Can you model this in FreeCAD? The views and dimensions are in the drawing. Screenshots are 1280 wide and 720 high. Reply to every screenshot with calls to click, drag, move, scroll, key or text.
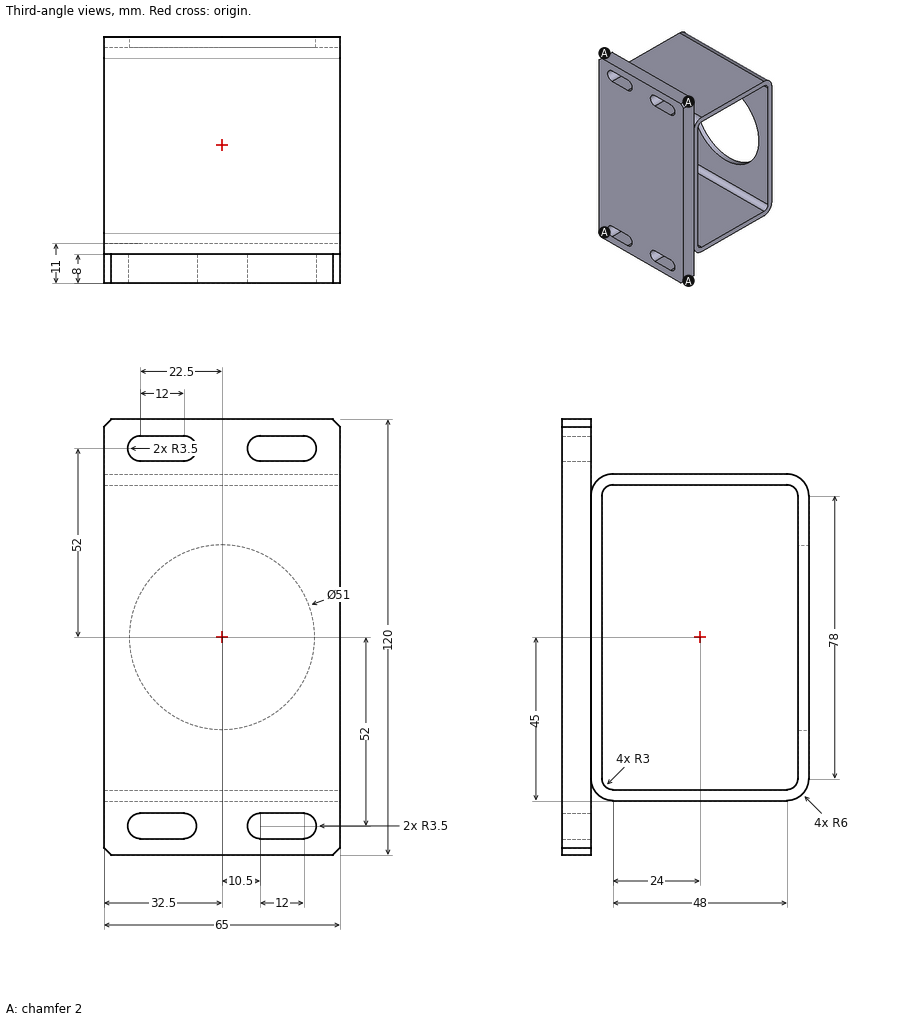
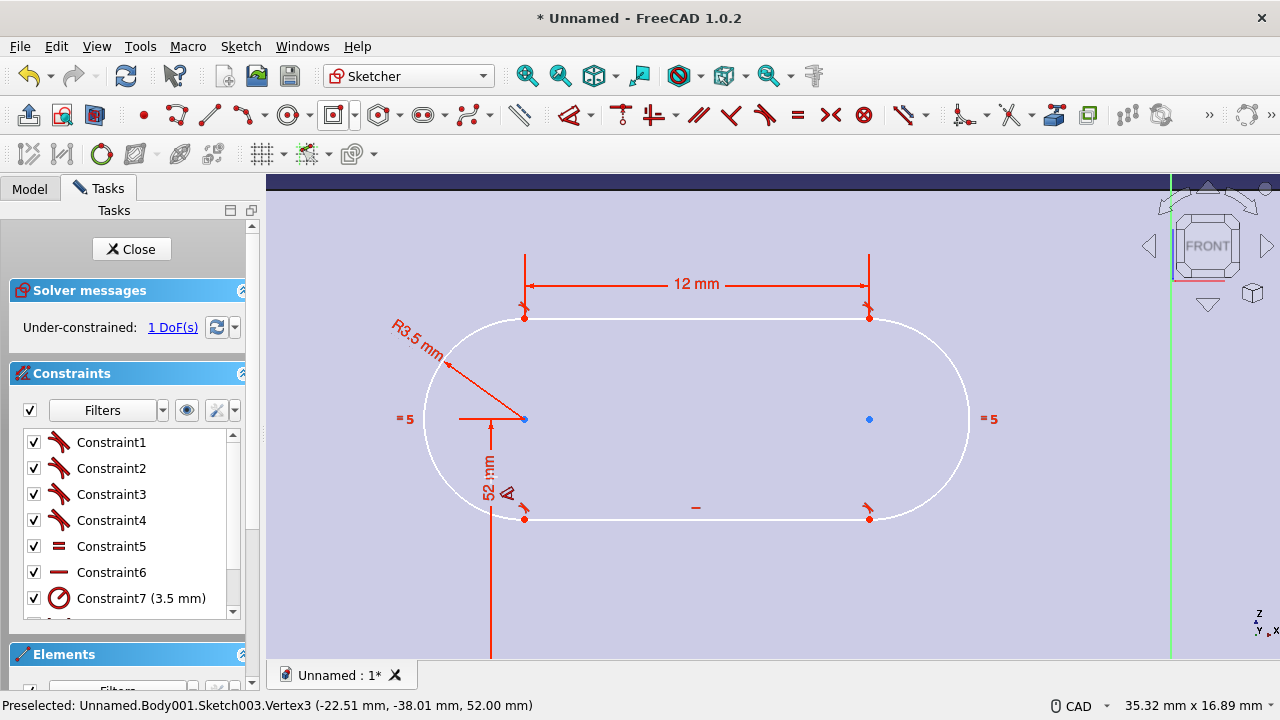
click(525, 319)
click(820, 285)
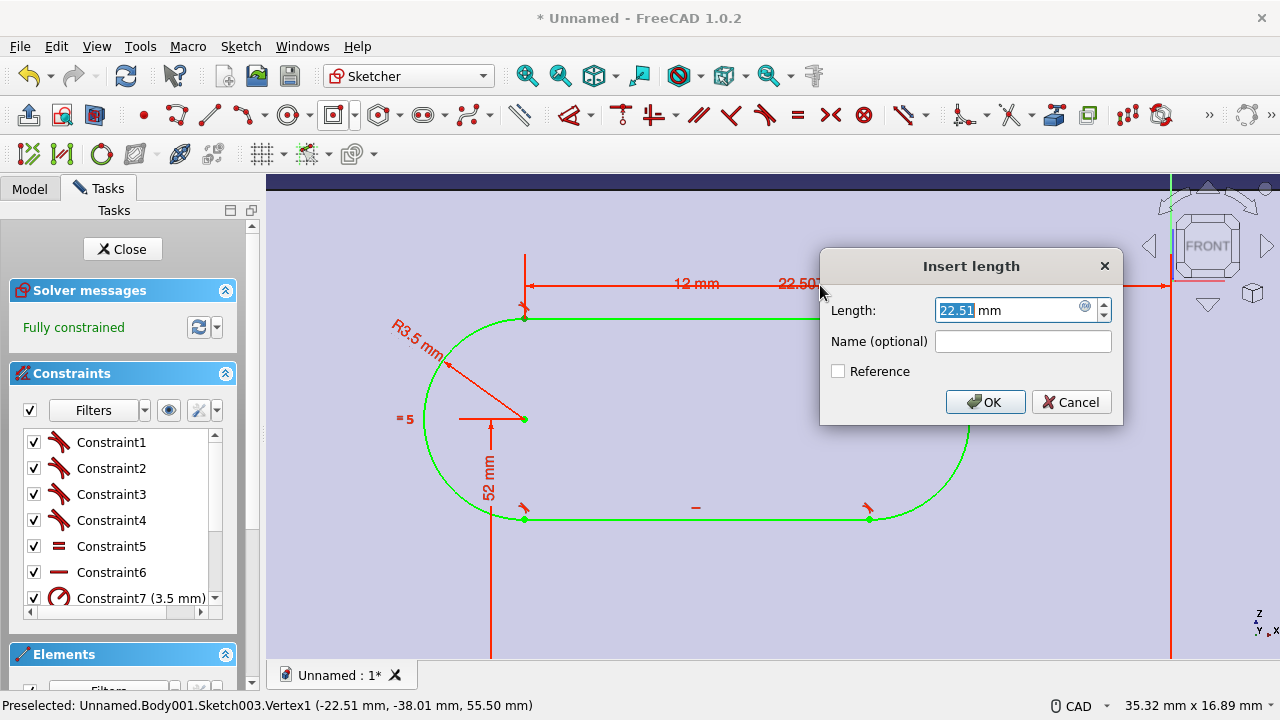
text(22.5)
key(Return)
key(Escape)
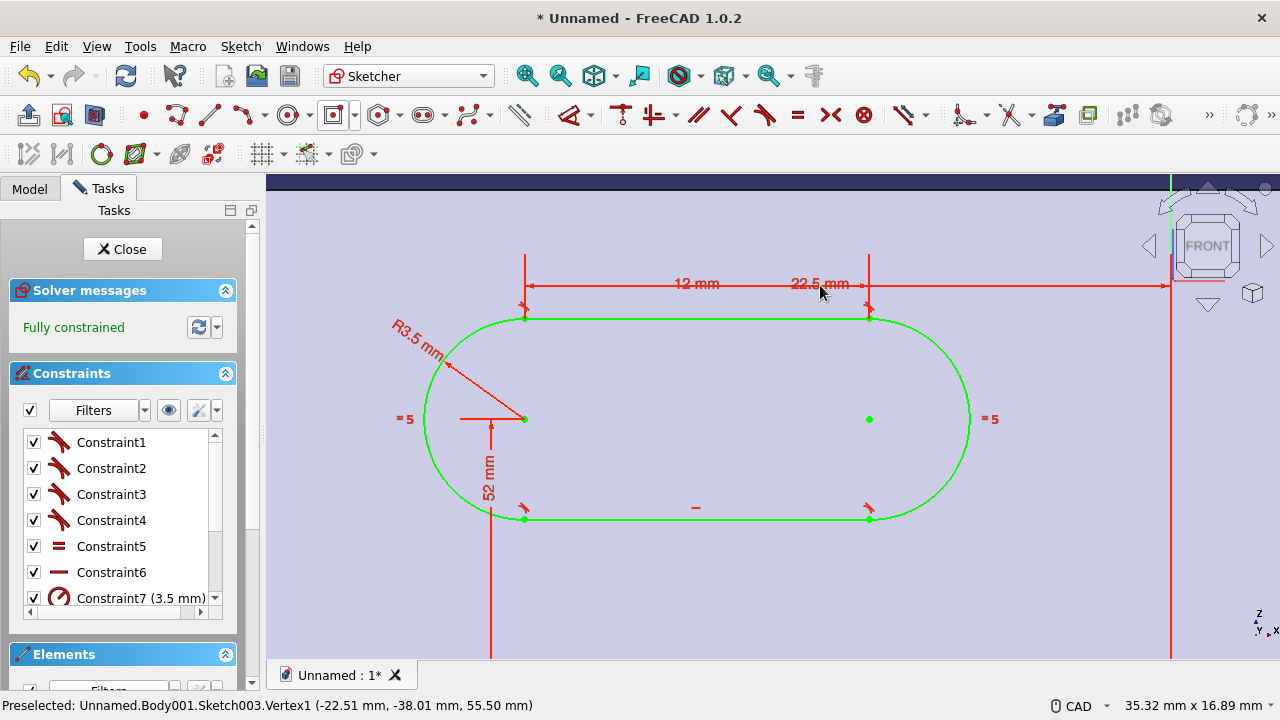
click(123, 249)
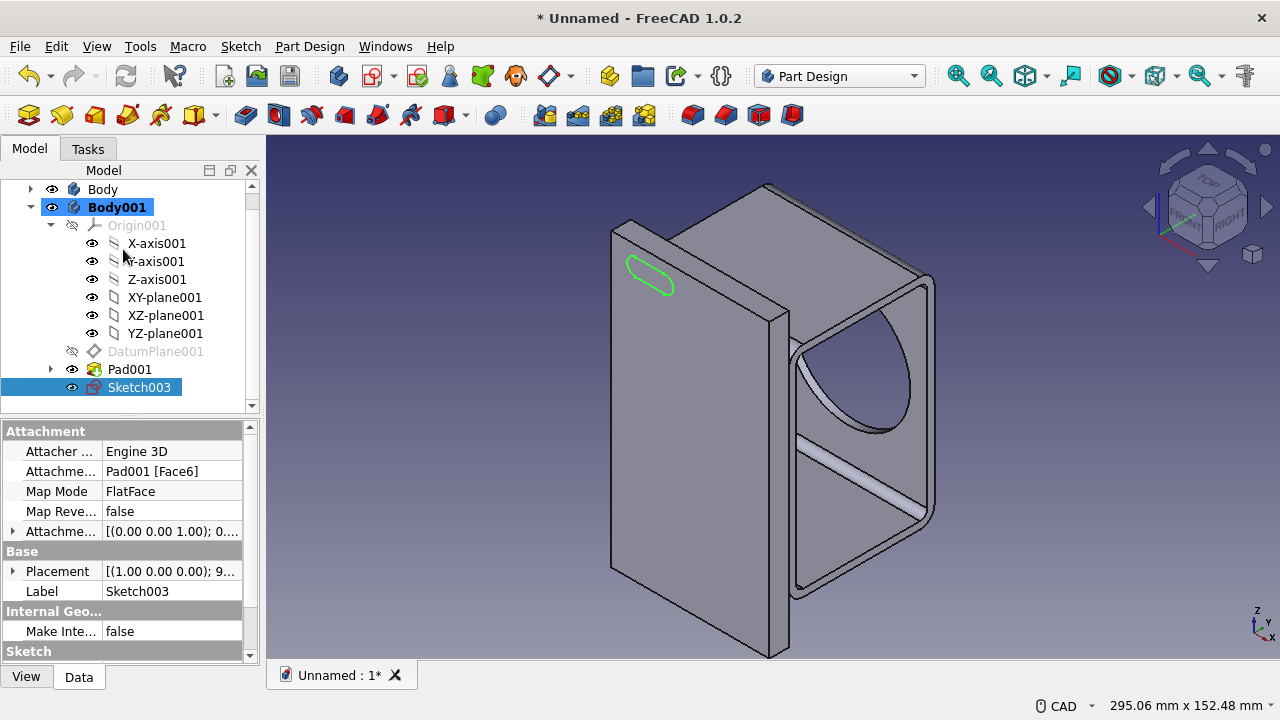
click(246, 116)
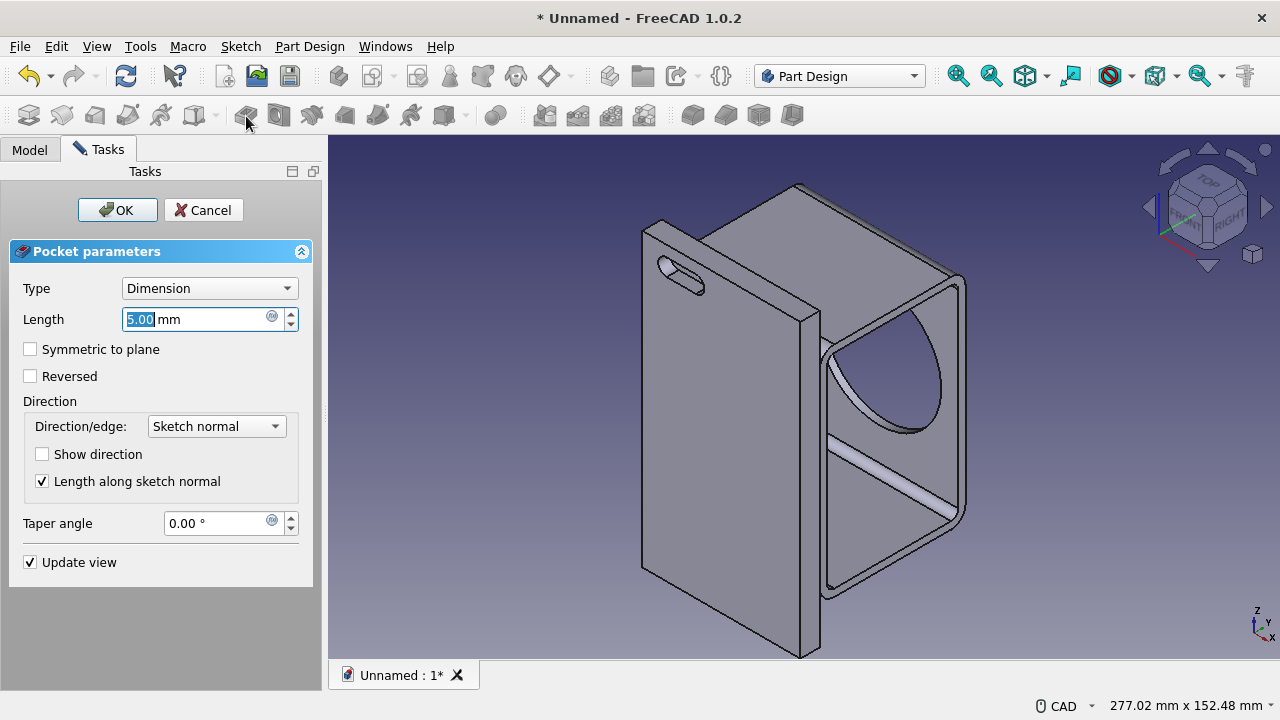
text(11)
key(Tab)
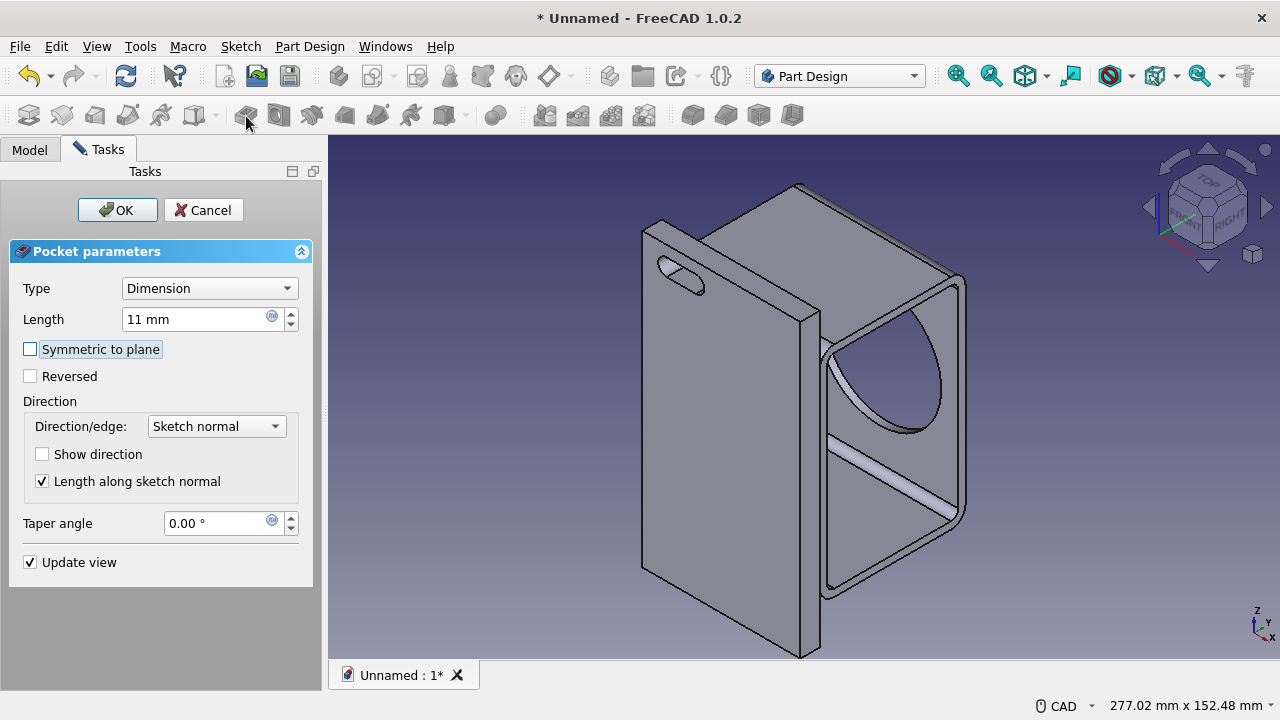
click(118, 210)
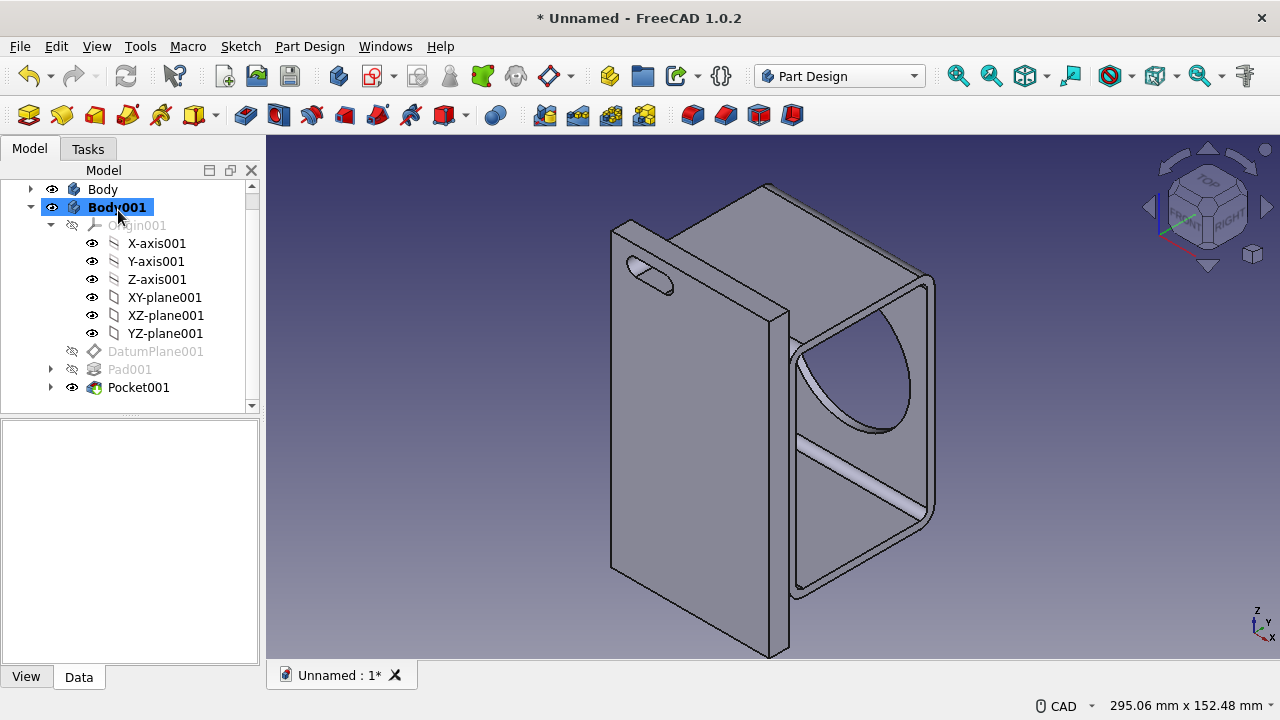
click(117, 387)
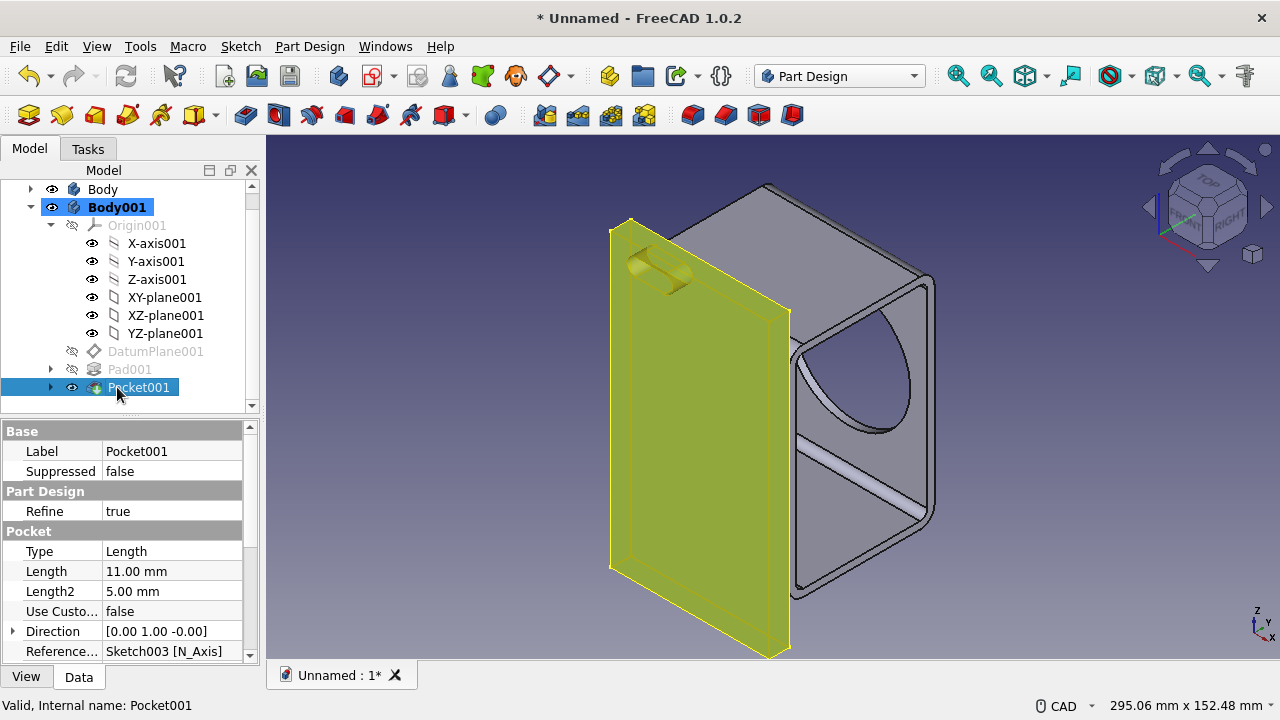
click(545, 116)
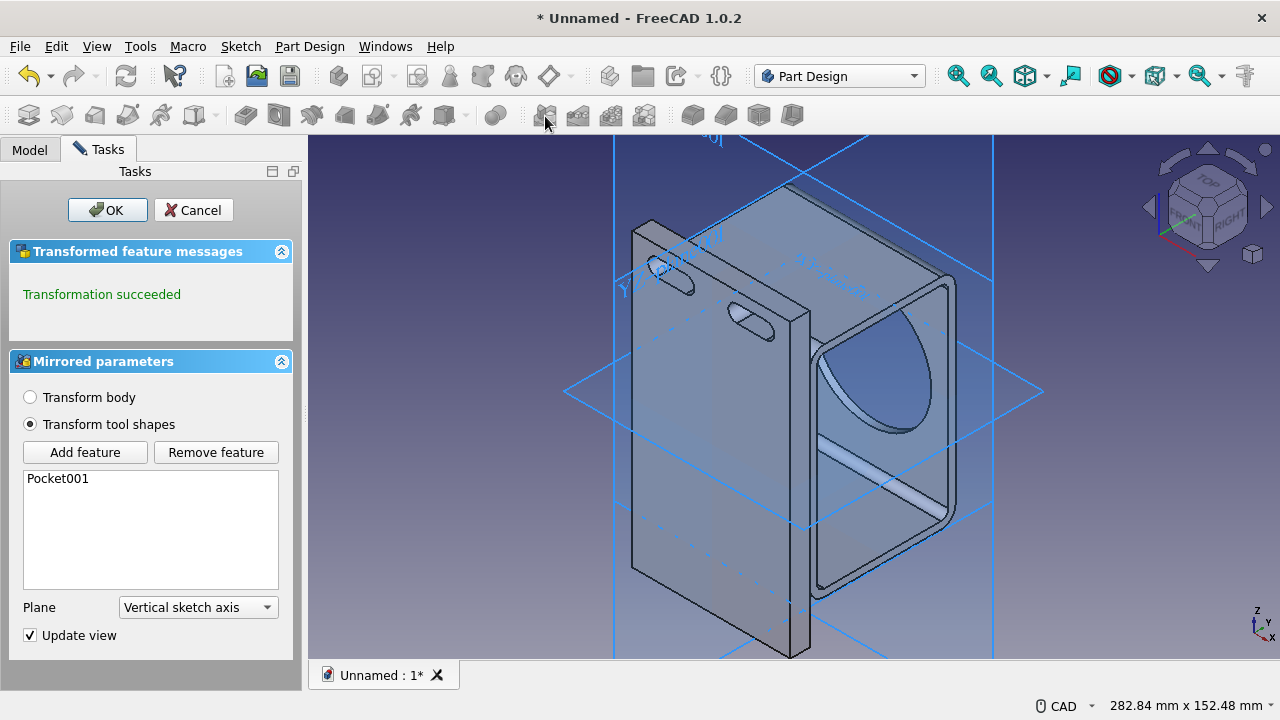
click(199, 608)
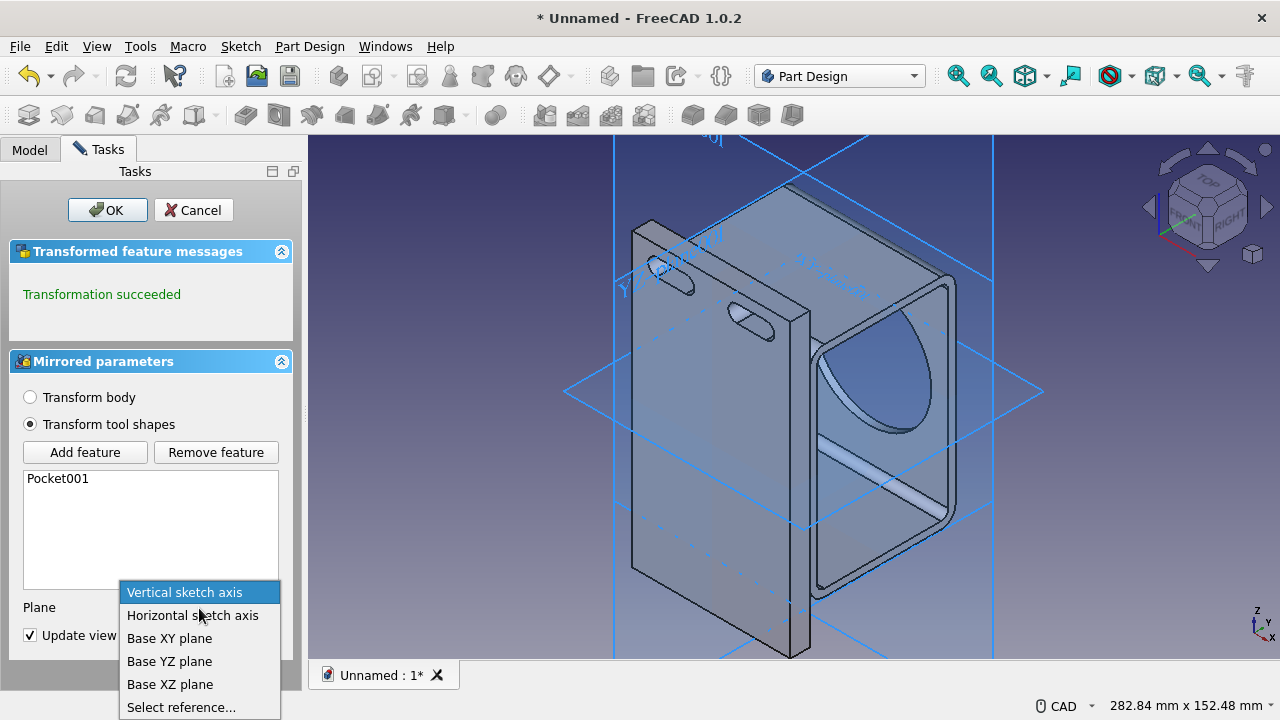
click(198, 662)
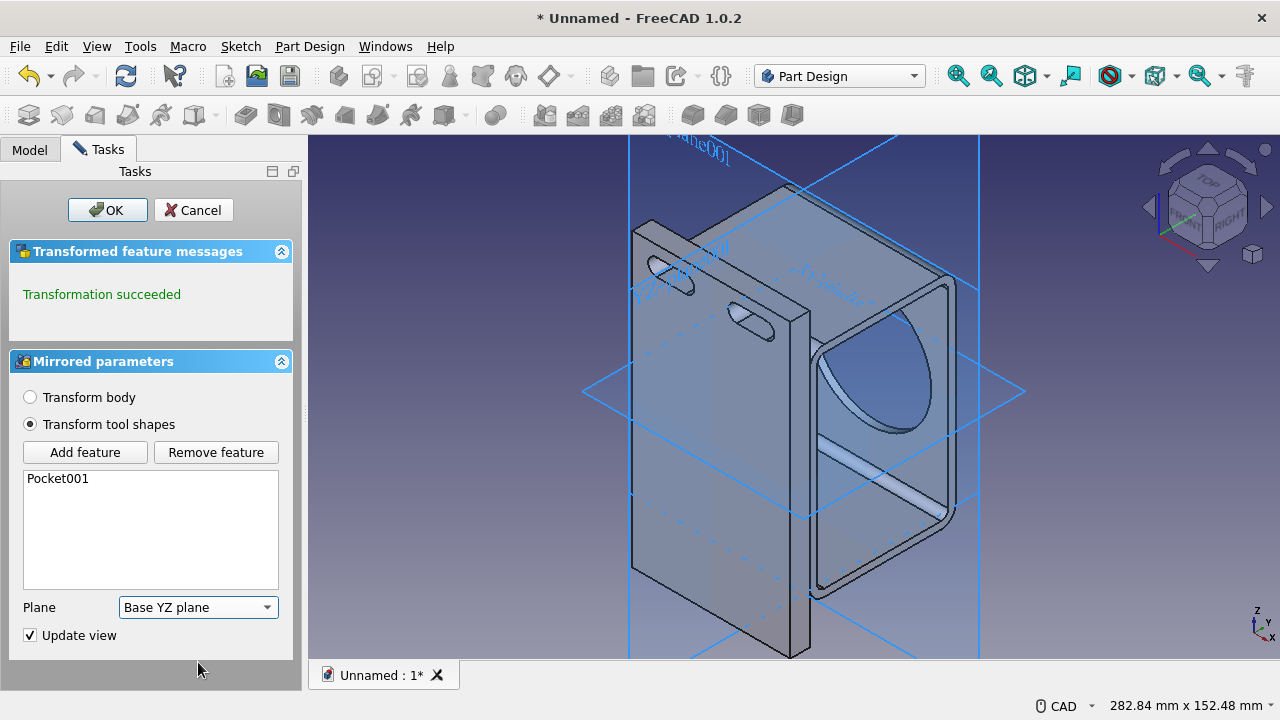
click(108, 210)